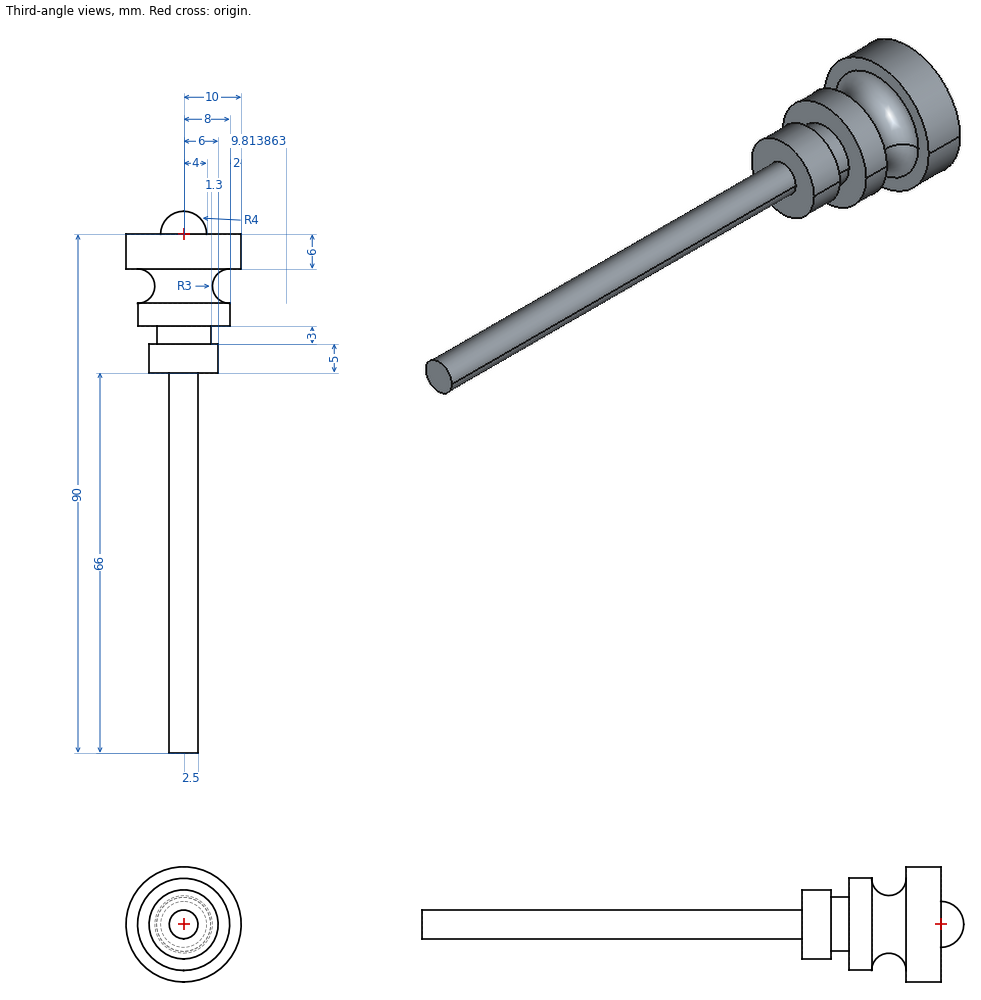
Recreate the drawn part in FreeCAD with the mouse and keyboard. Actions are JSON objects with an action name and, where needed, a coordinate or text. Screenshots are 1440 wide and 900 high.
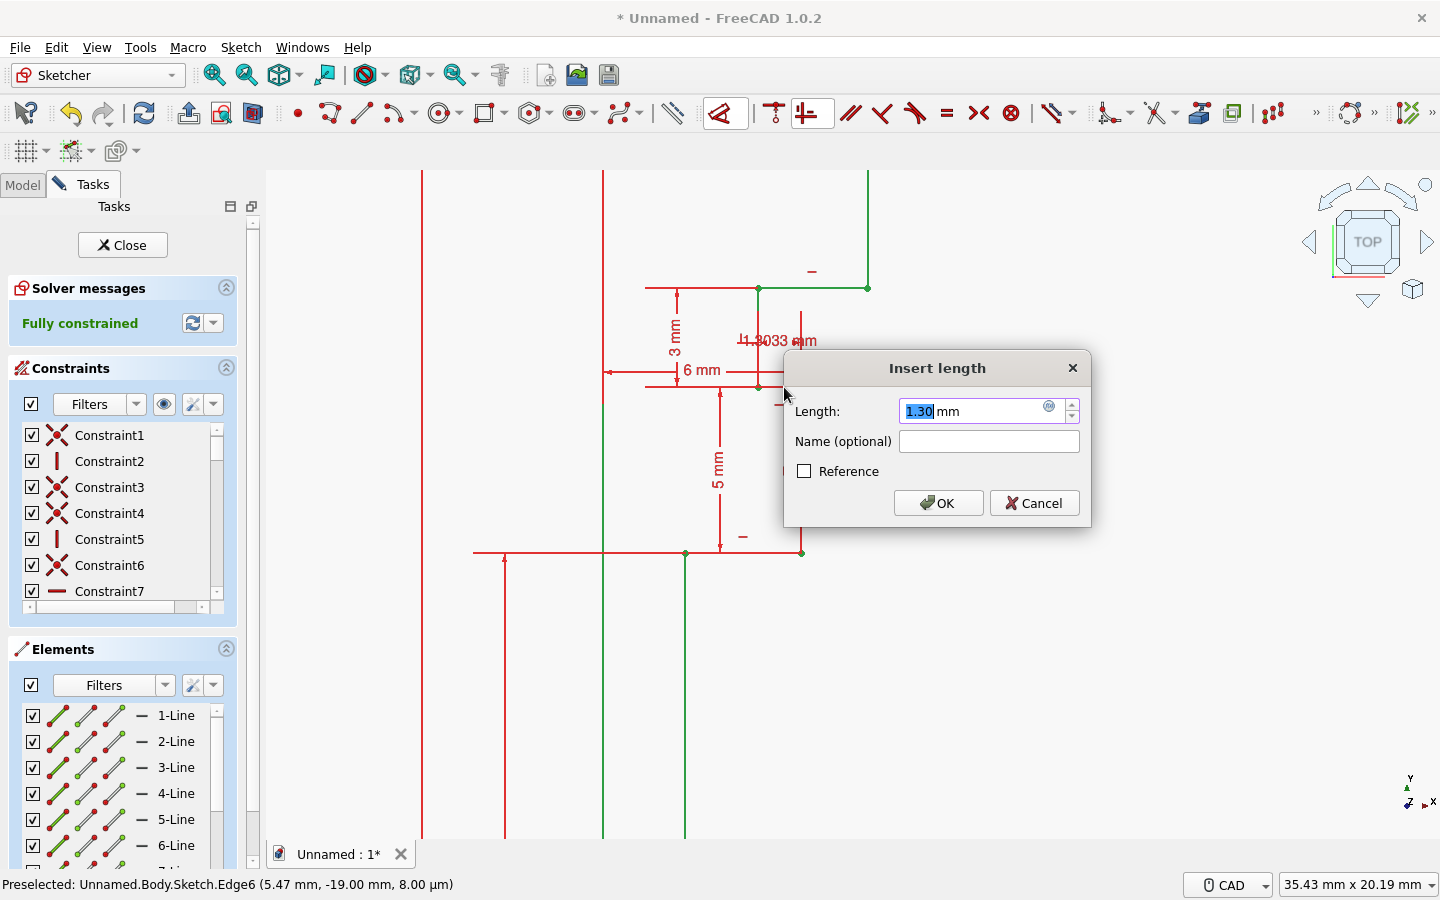
{"action": "type", "text": "1.3"}
{"action": "key", "text": "Return"}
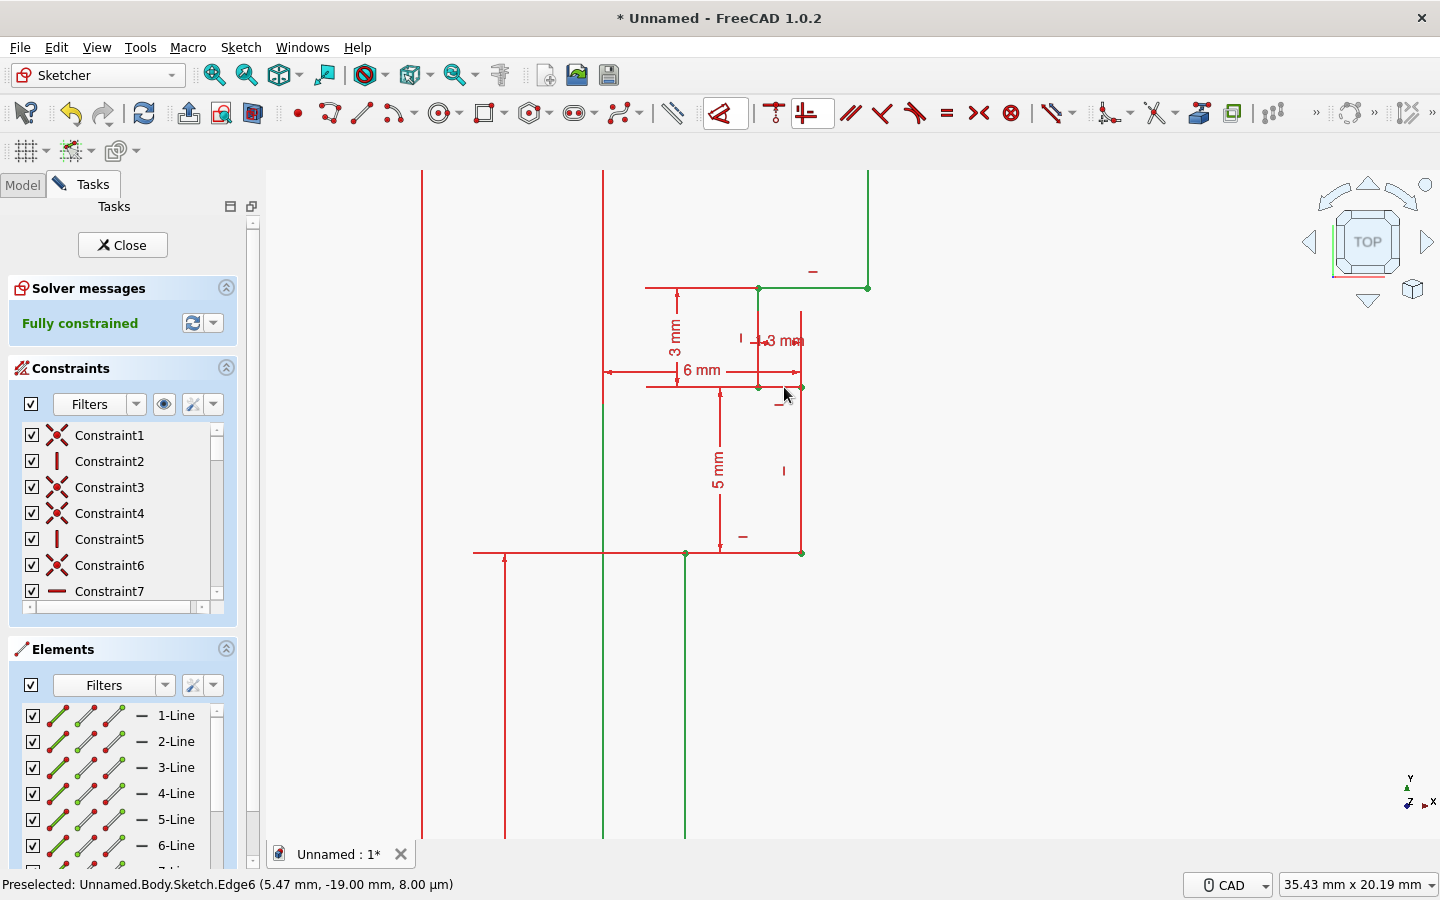
{"action": "left_click", "coordinate": [123, 245]}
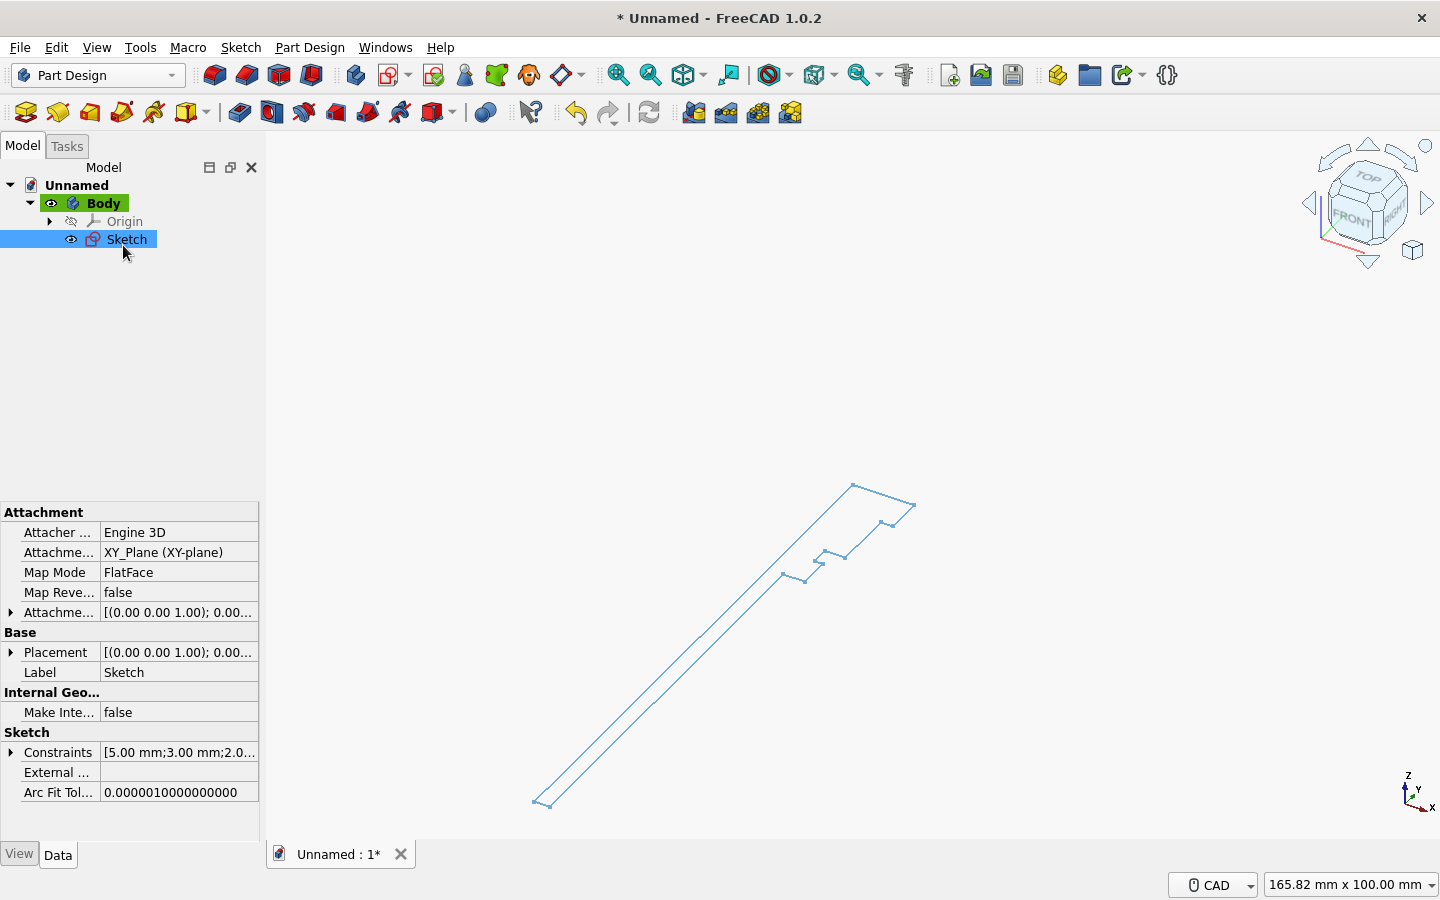
{"action": "left_click", "coordinate": [58, 112]}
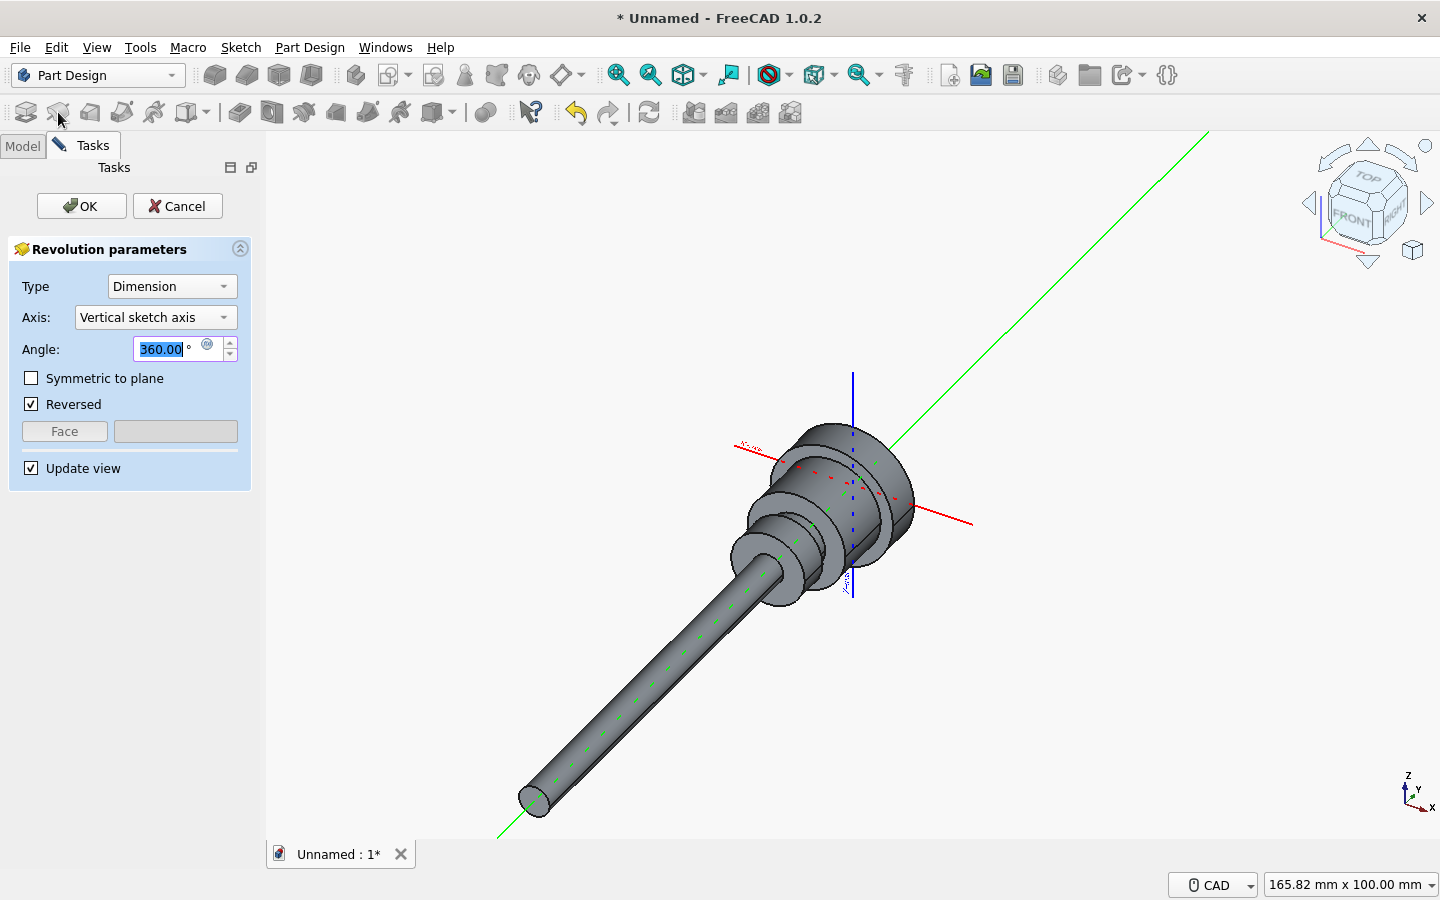
{"action": "left_click", "coordinate": [82, 206]}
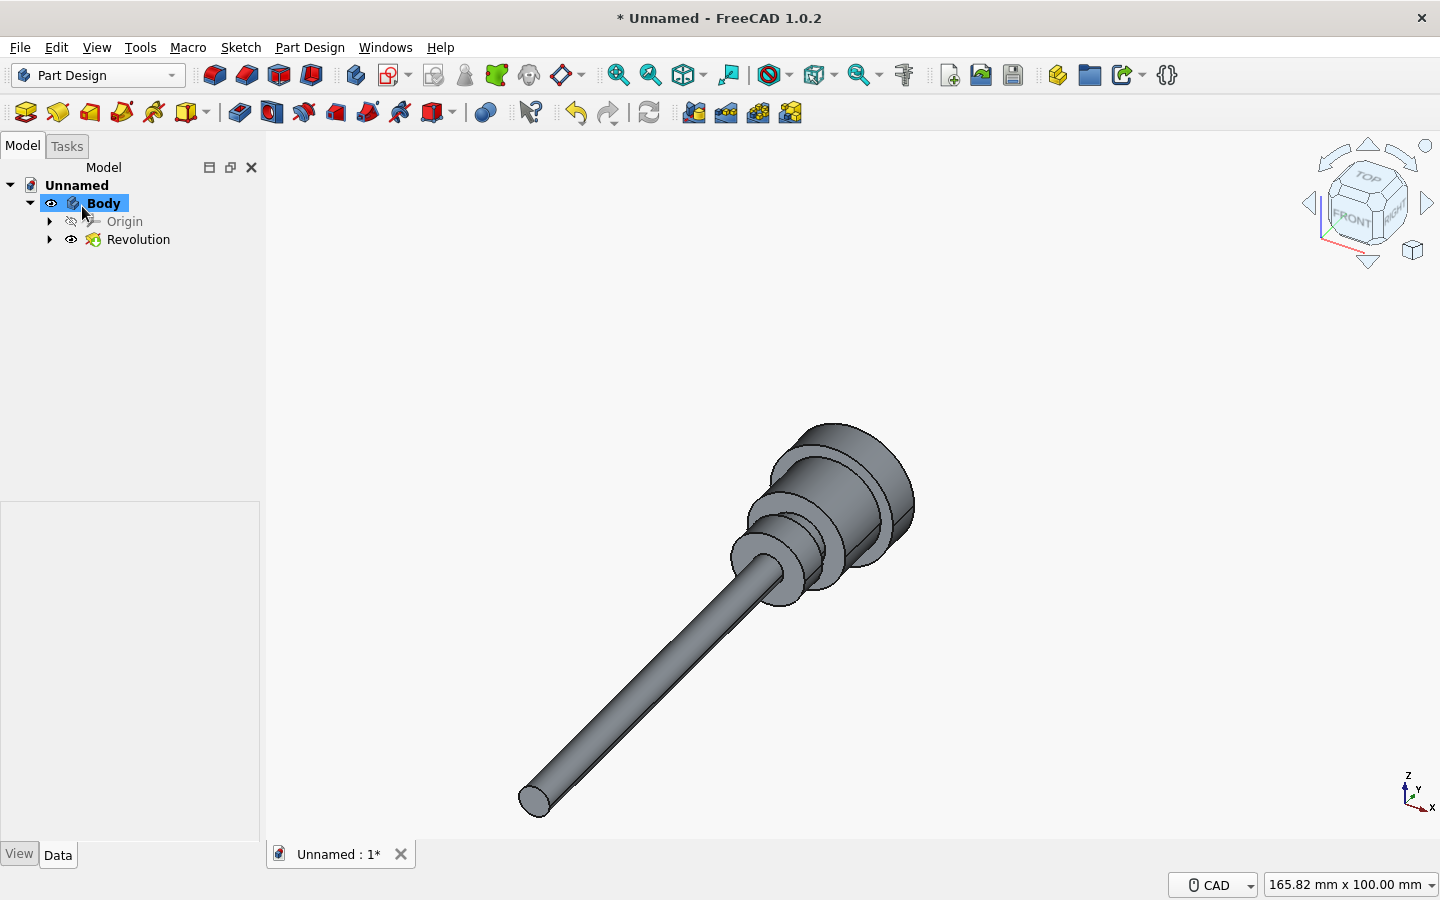
{"action": "left_click", "coordinate": [620, 76]}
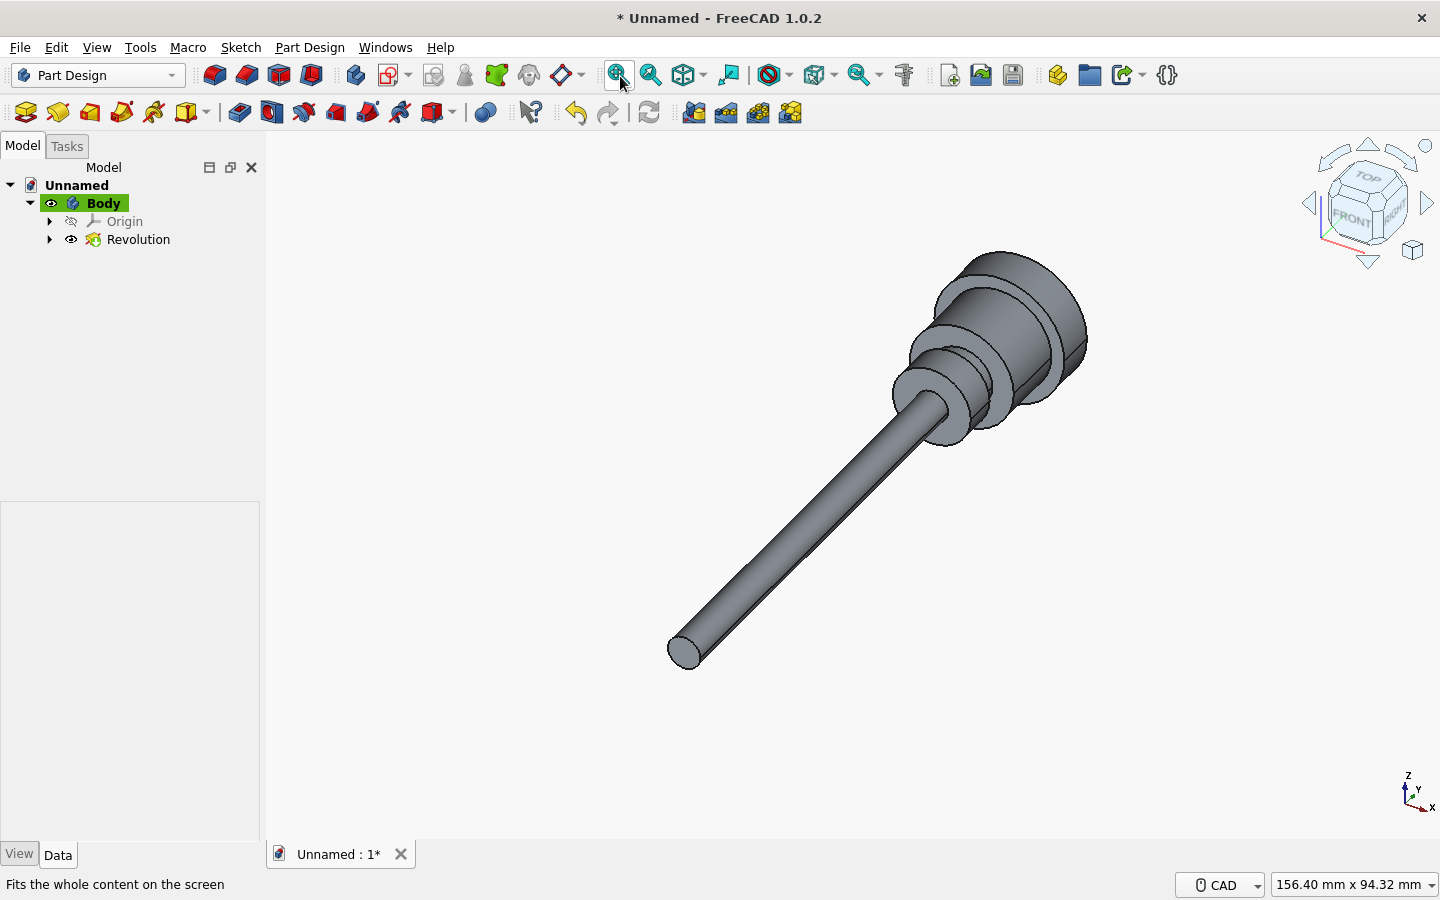
{"action": "left_click", "coordinate": [388, 76]}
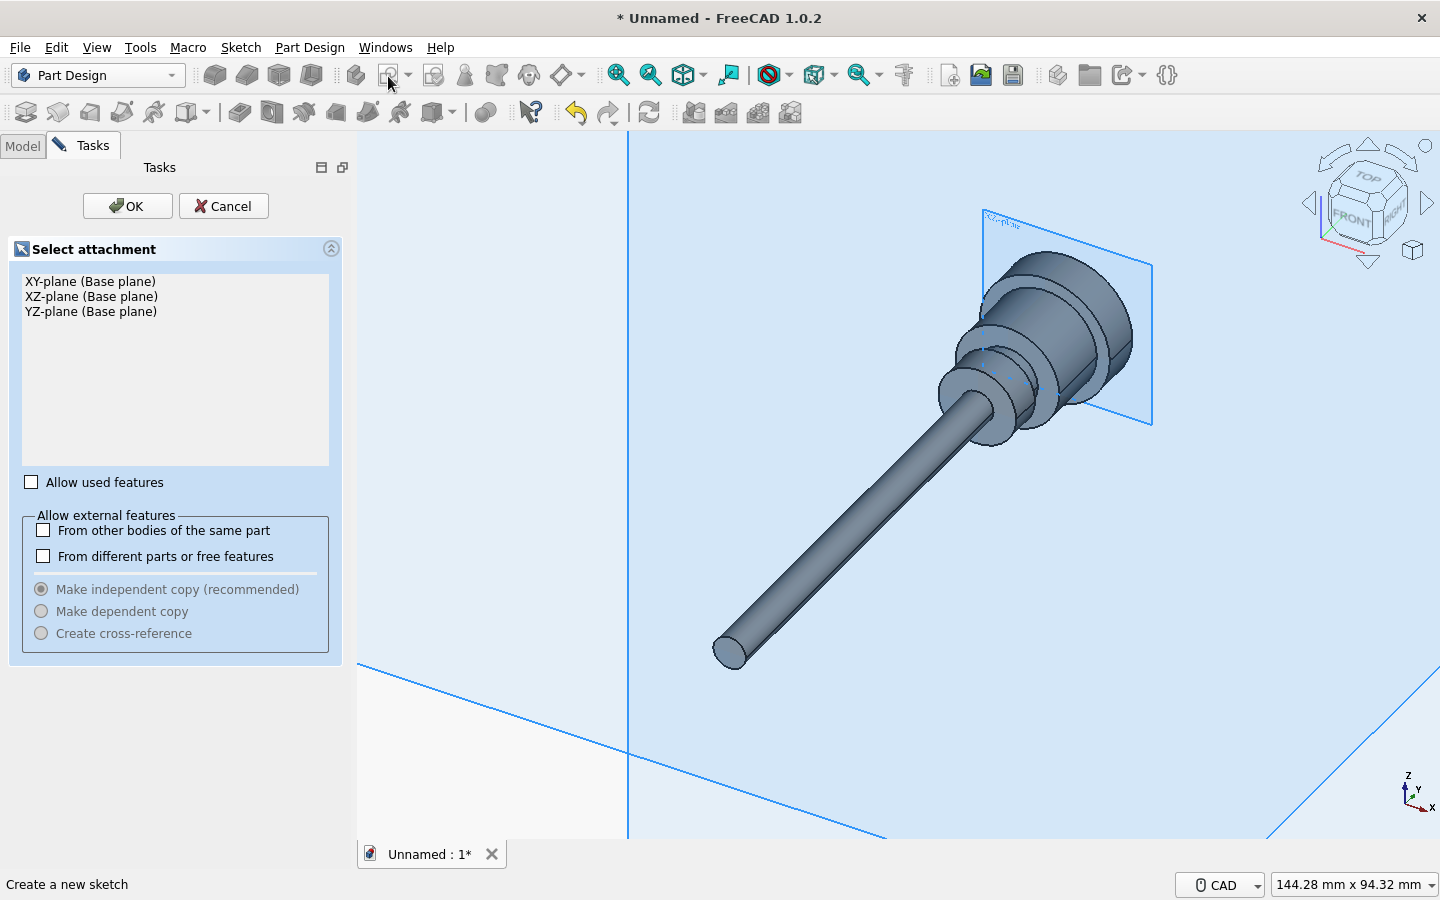
{"action": "left_click", "coordinate": [82, 282]}